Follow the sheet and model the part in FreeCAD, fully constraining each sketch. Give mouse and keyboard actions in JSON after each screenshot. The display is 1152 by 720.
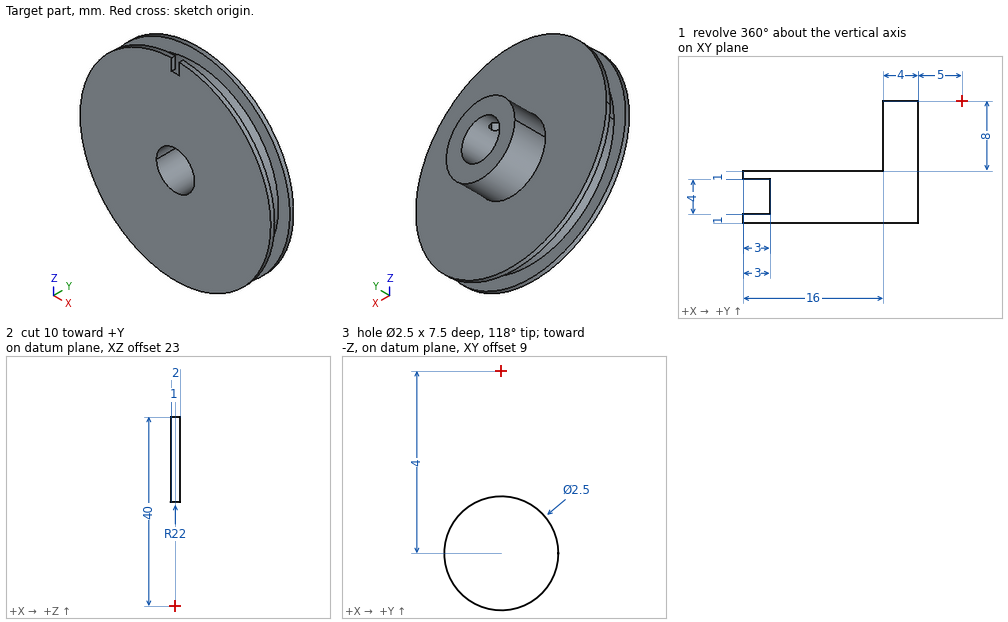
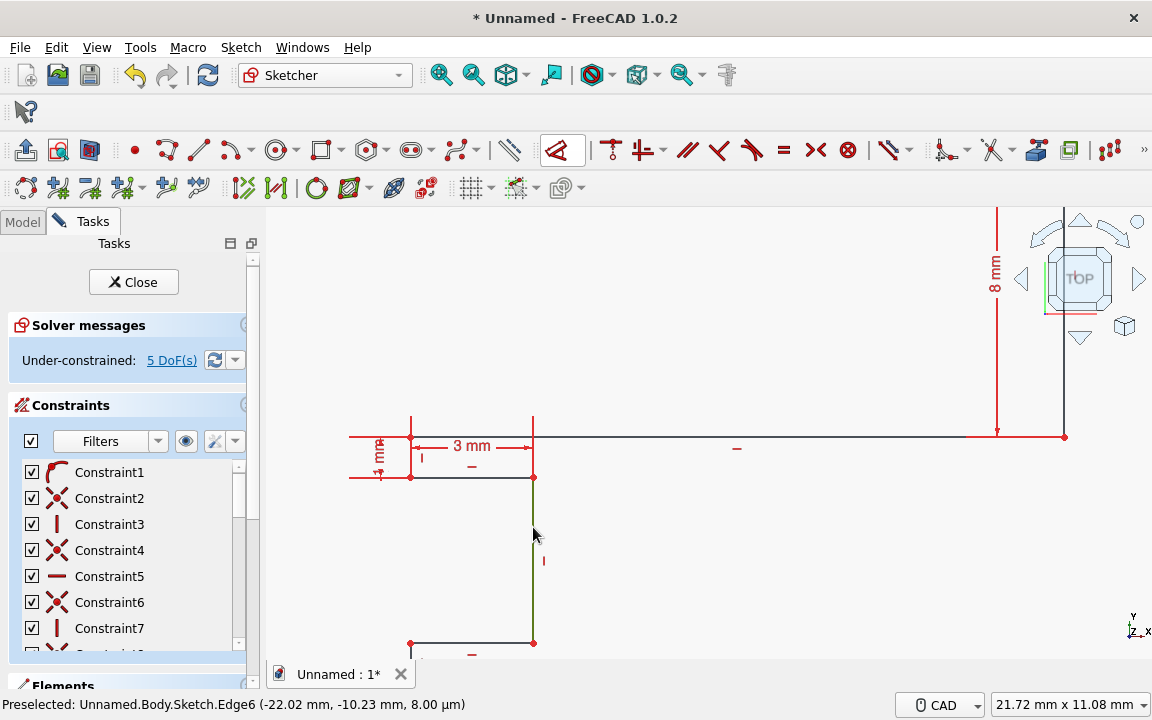
{"action": "key", "text": "i"}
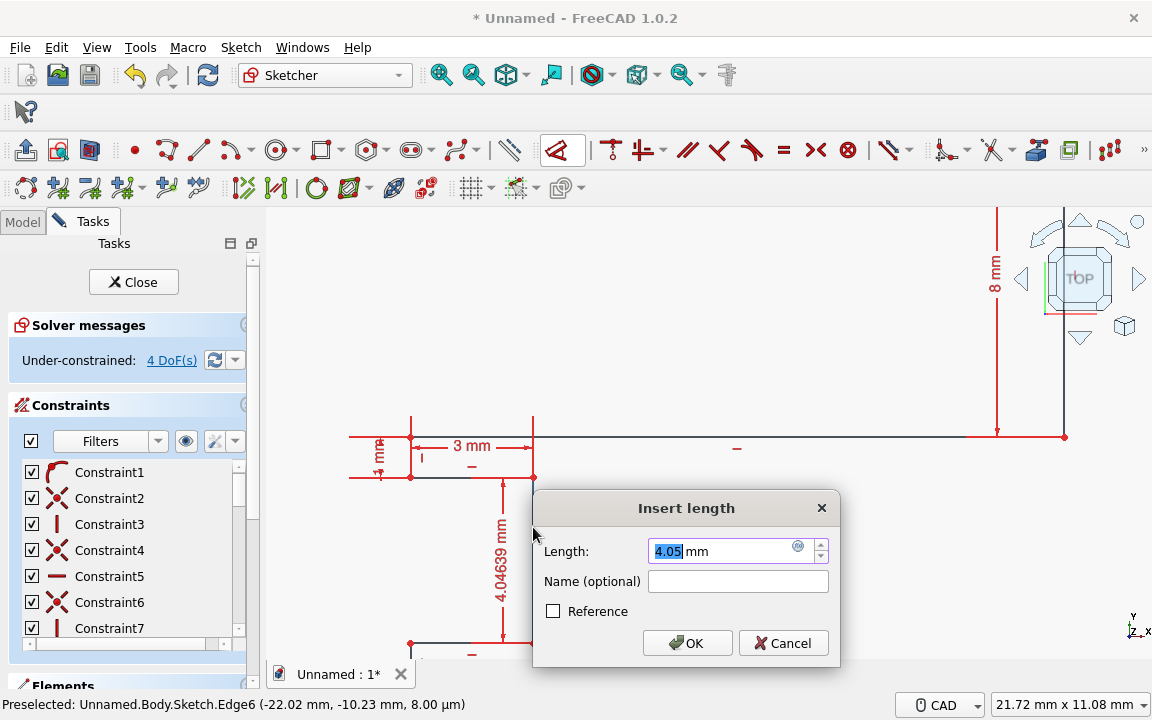
{"action": "type", "text": "4"}
{"action": "key", "text": "Return"}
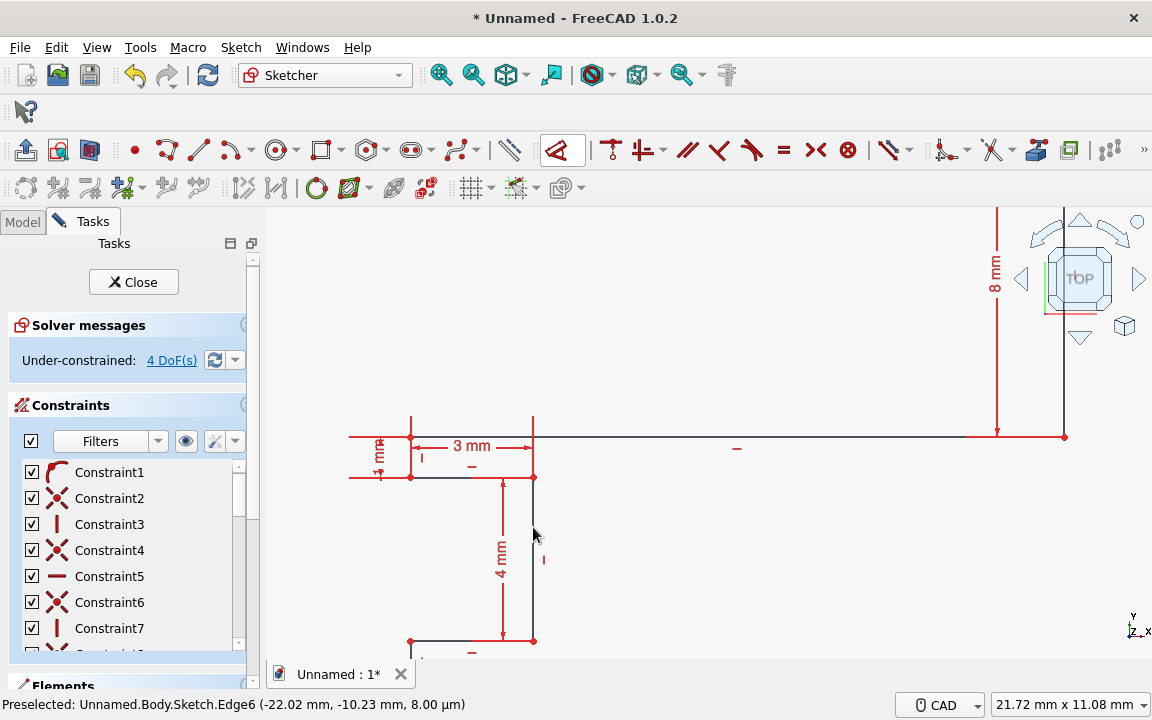
{"action": "scroll", "coordinate": [411, 463], "scroll_direction": "down", "scroll_amount": 4}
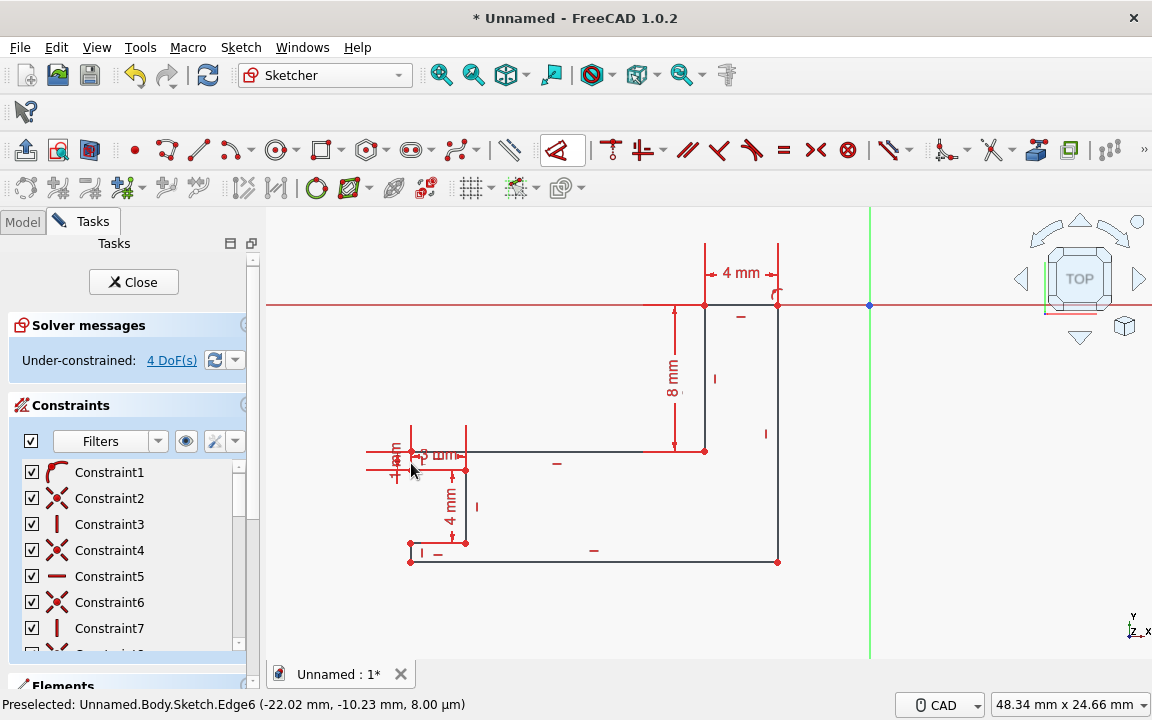
{"action": "left_click", "coordinate": [449, 543]}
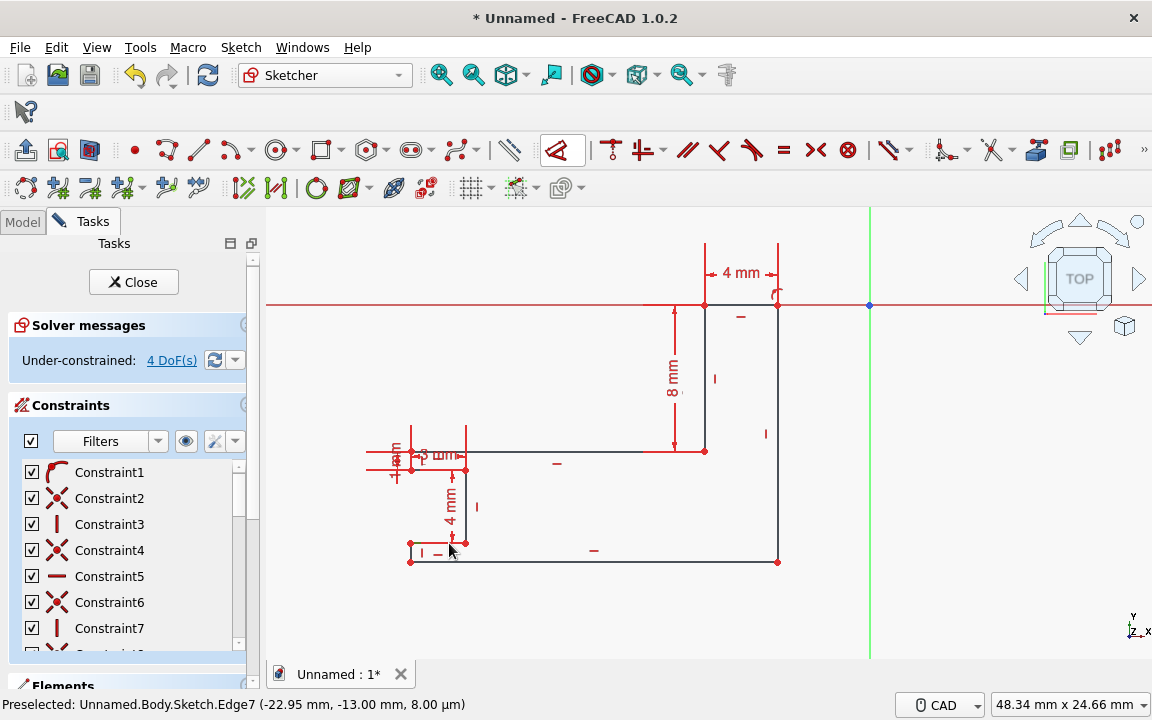
{"action": "key", "text": "l"}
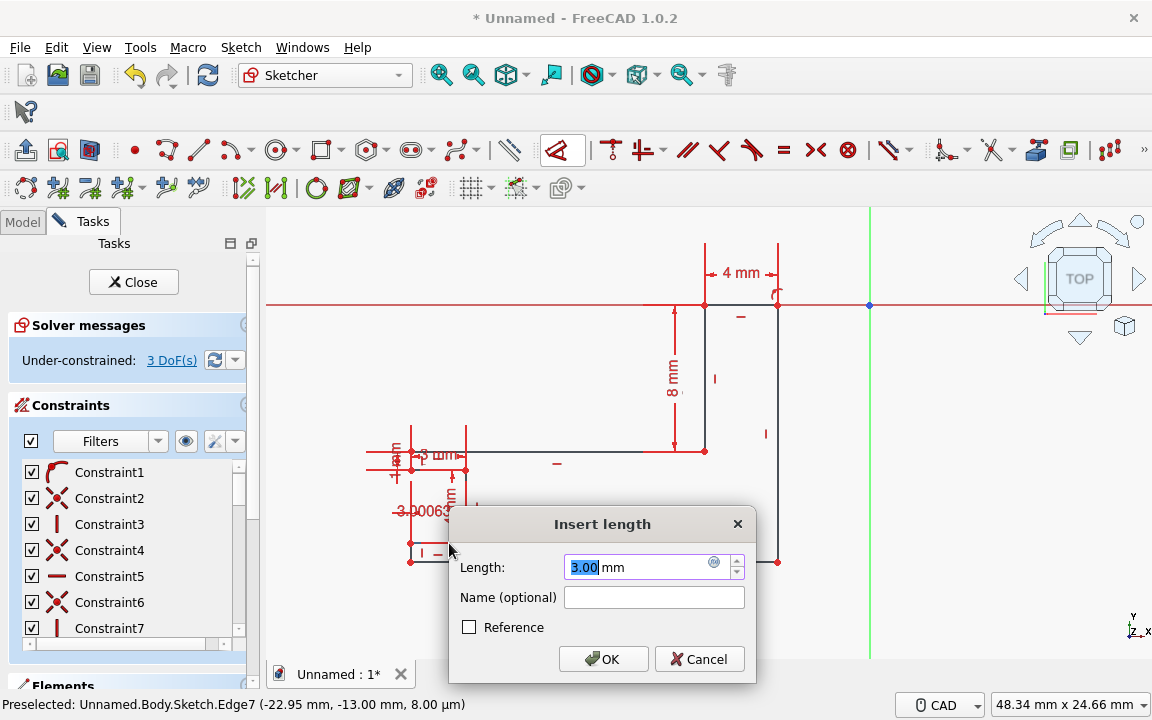
{"action": "type", "text": "3"}
{"action": "key", "text": "Return"}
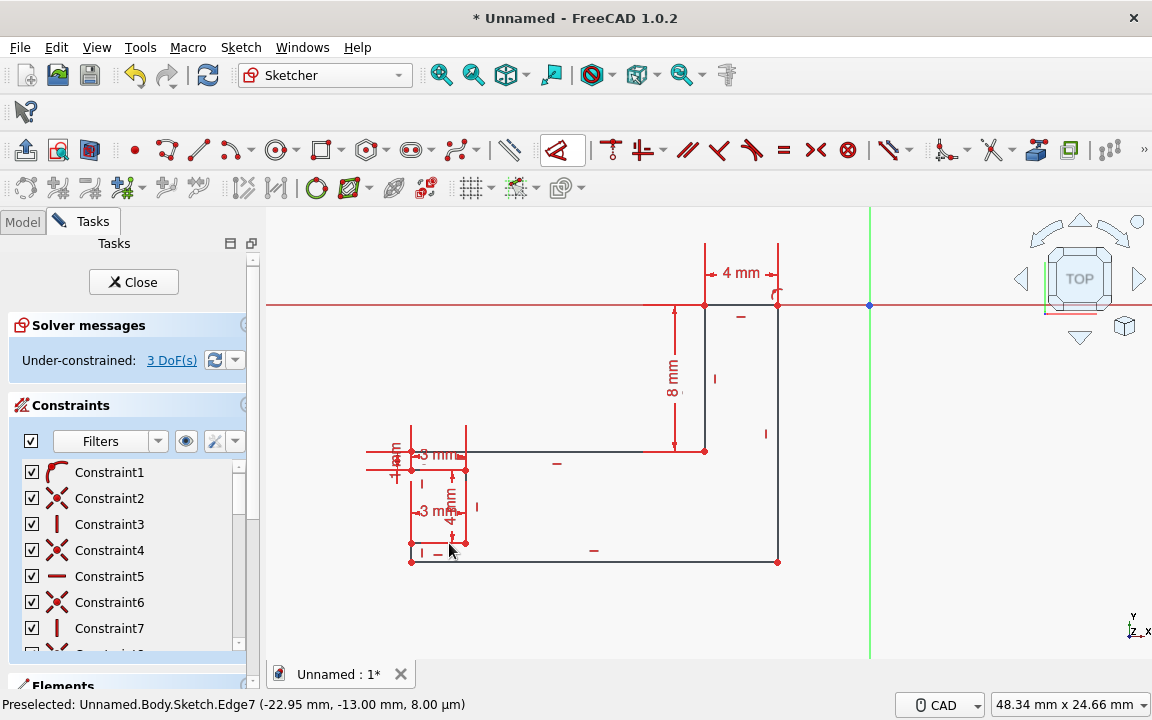
{"action": "scroll", "coordinate": [411, 553], "scroll_direction": "up", "scroll_amount": 4}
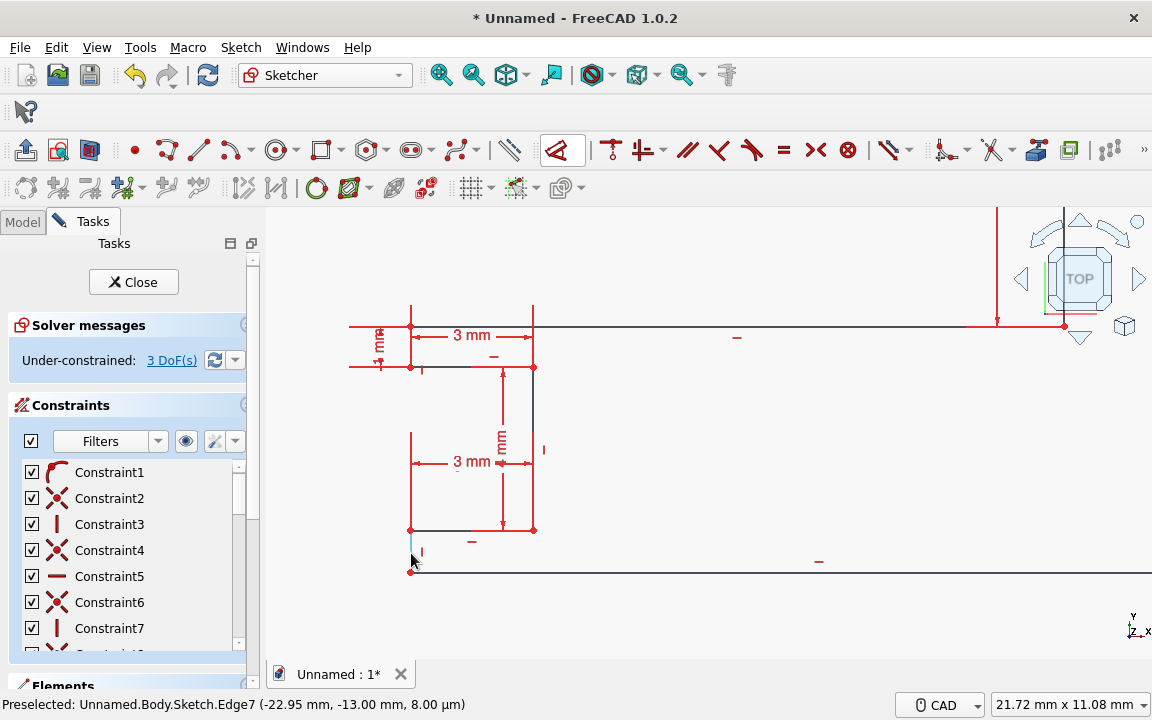
{"action": "left_click", "coordinate": [411, 552]}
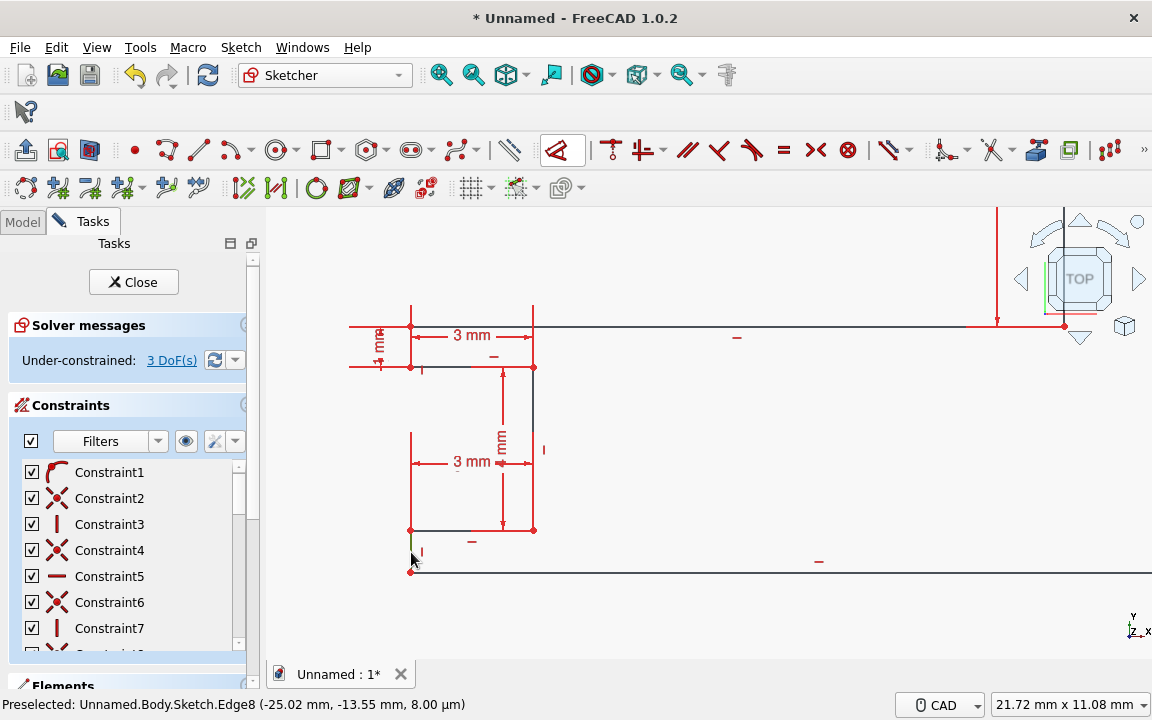
{"action": "key", "text": "i"}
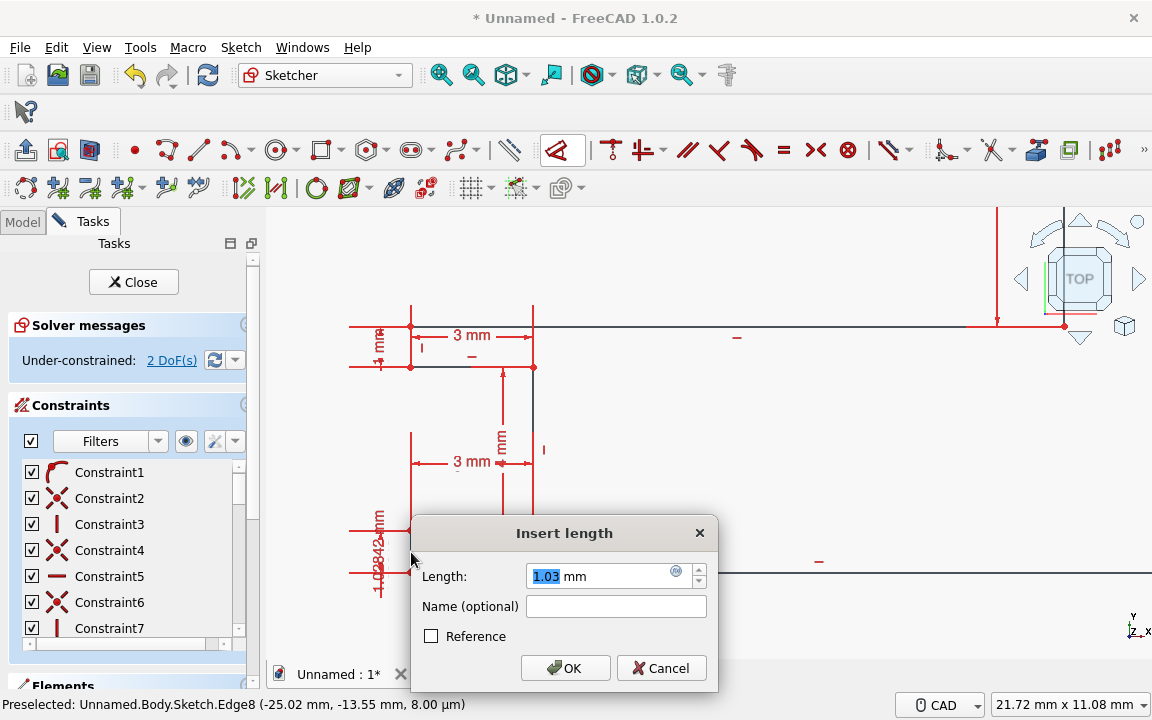
{"action": "type", "text": "1"}
{"action": "key", "text": "Return"}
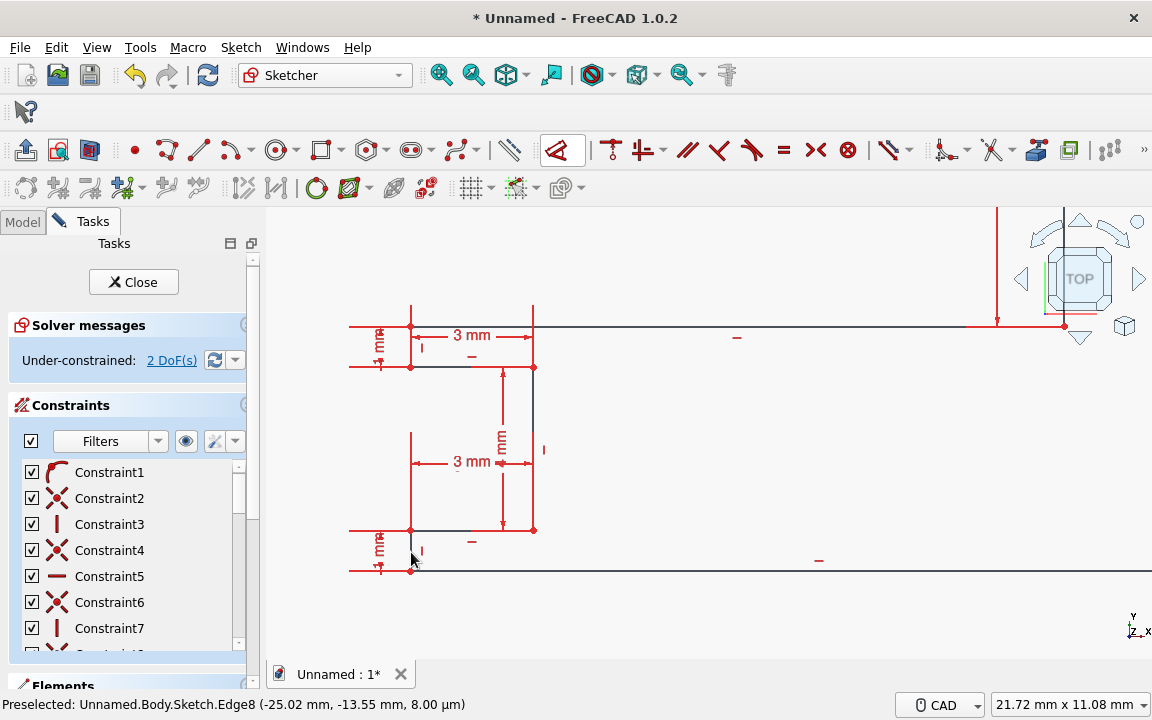
{"action": "left_click", "coordinate": [868, 327]}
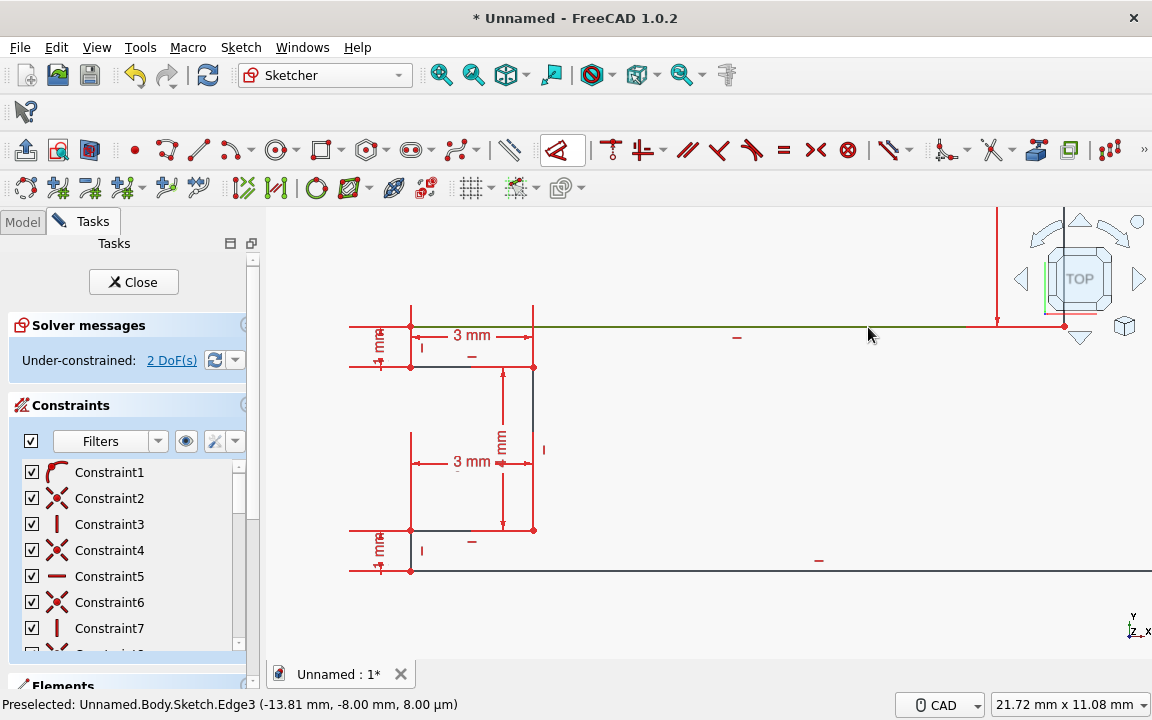
{"action": "key", "text": "l"}